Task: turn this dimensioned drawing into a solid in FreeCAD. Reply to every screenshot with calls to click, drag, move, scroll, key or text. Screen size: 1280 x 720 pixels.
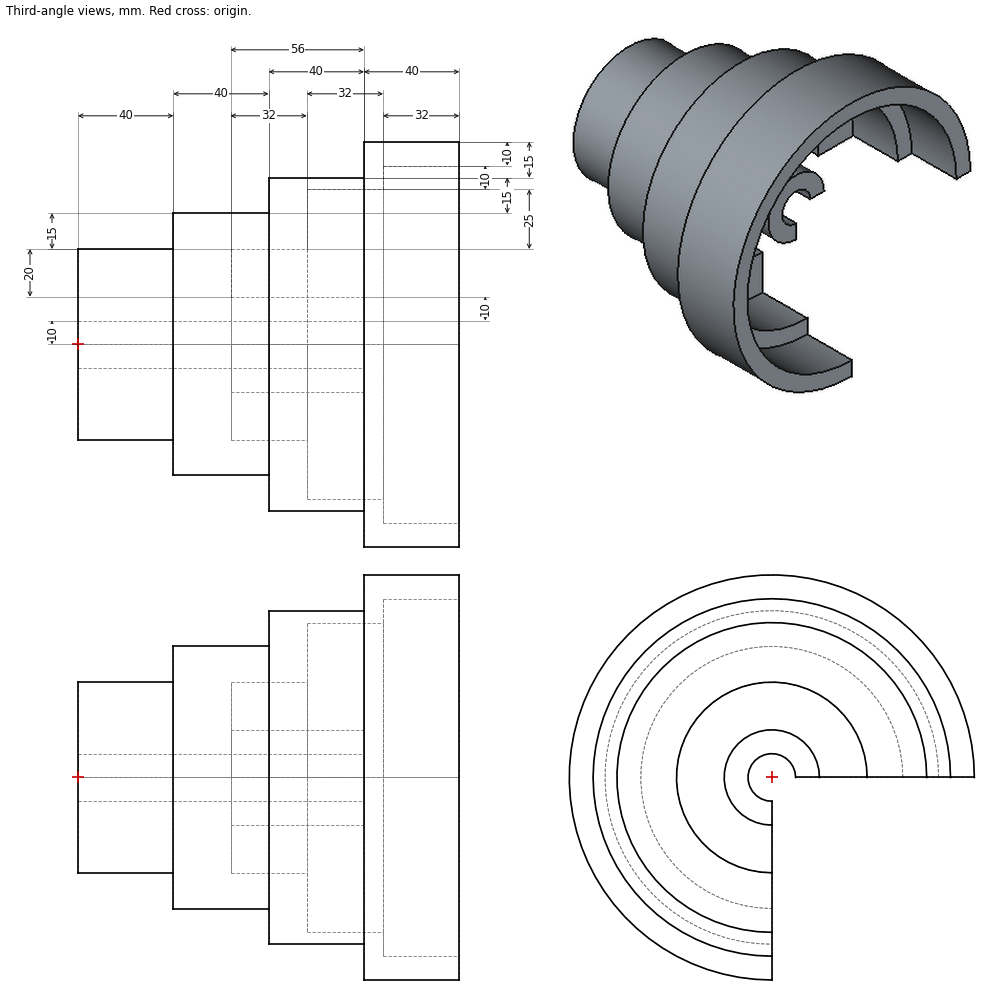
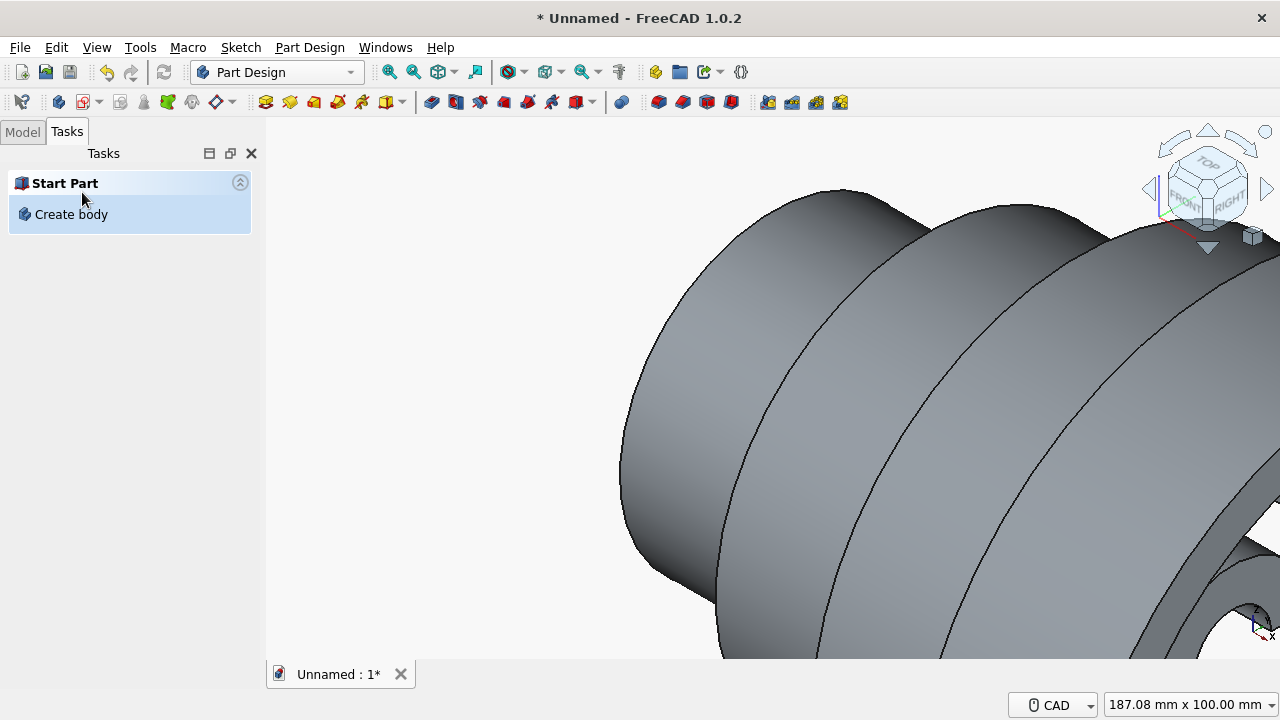
key(v)
key(f)